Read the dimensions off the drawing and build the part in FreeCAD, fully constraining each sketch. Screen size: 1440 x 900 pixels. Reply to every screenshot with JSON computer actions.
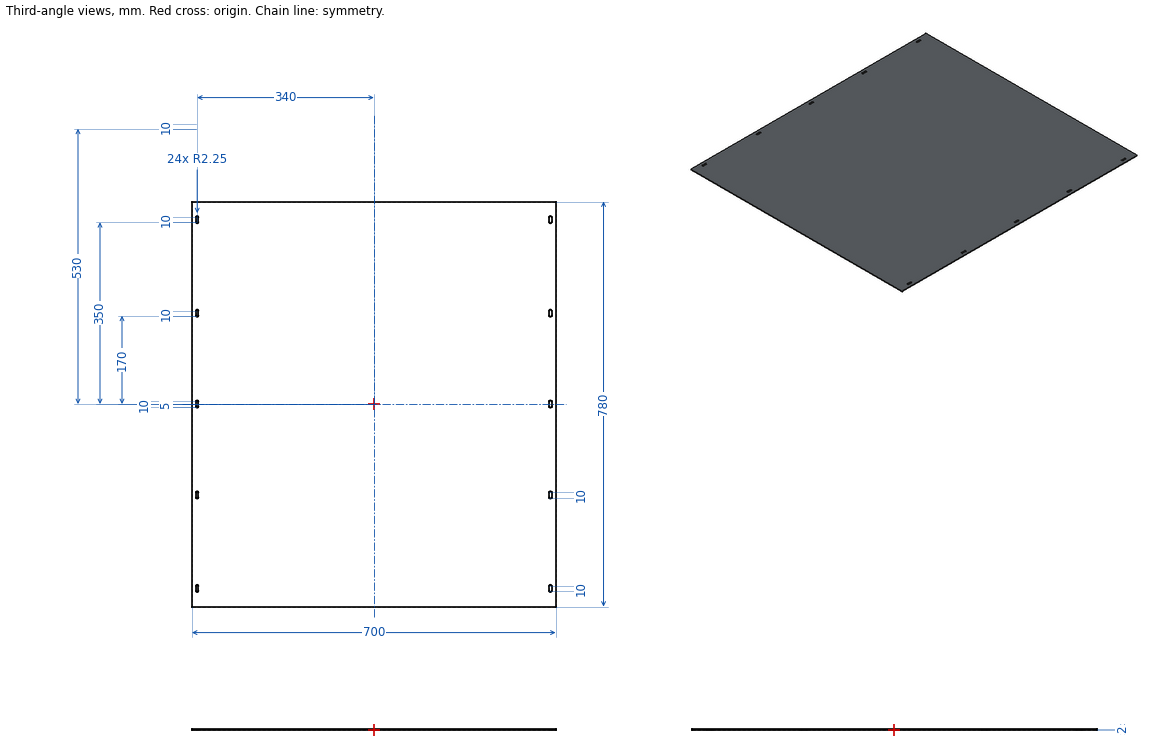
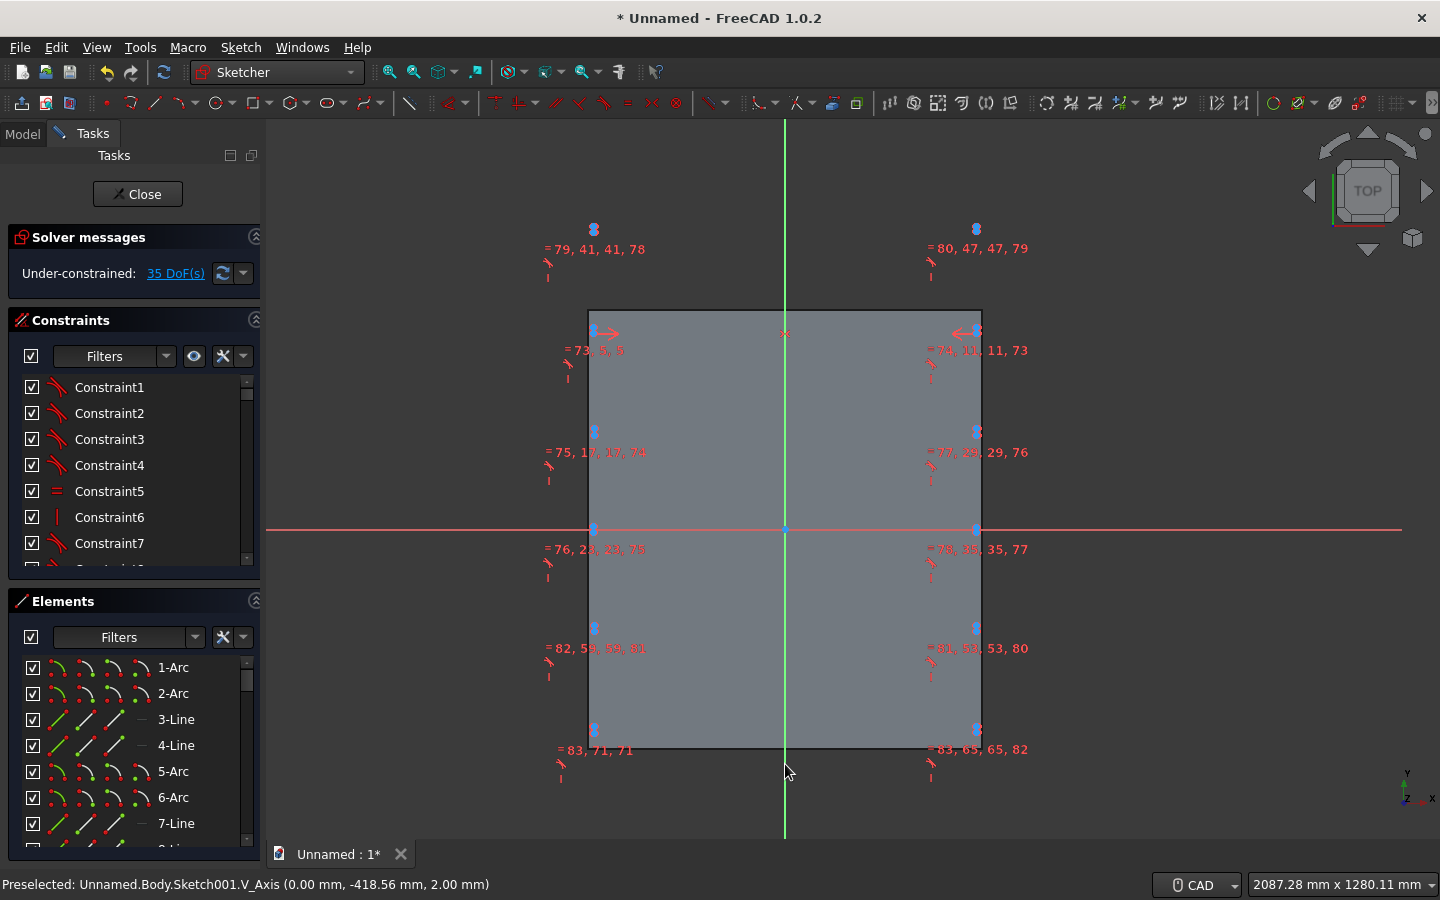
{"action": "scroll", "coordinate": [594, 435], "scroll_direction": "up", "scroll_amount": 12}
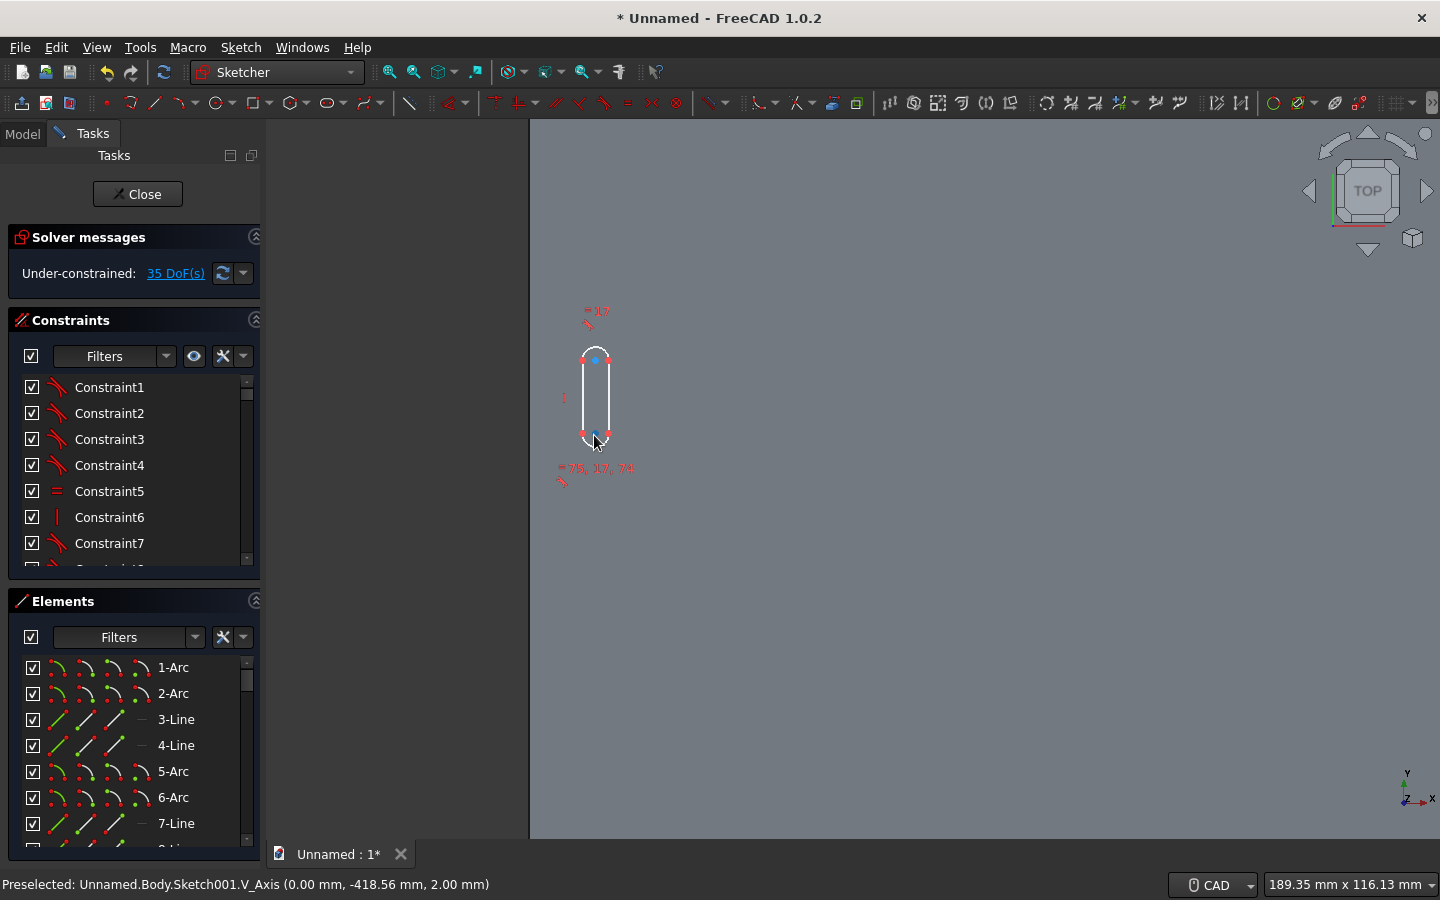
{"action": "left_click", "coordinate": [596, 434]}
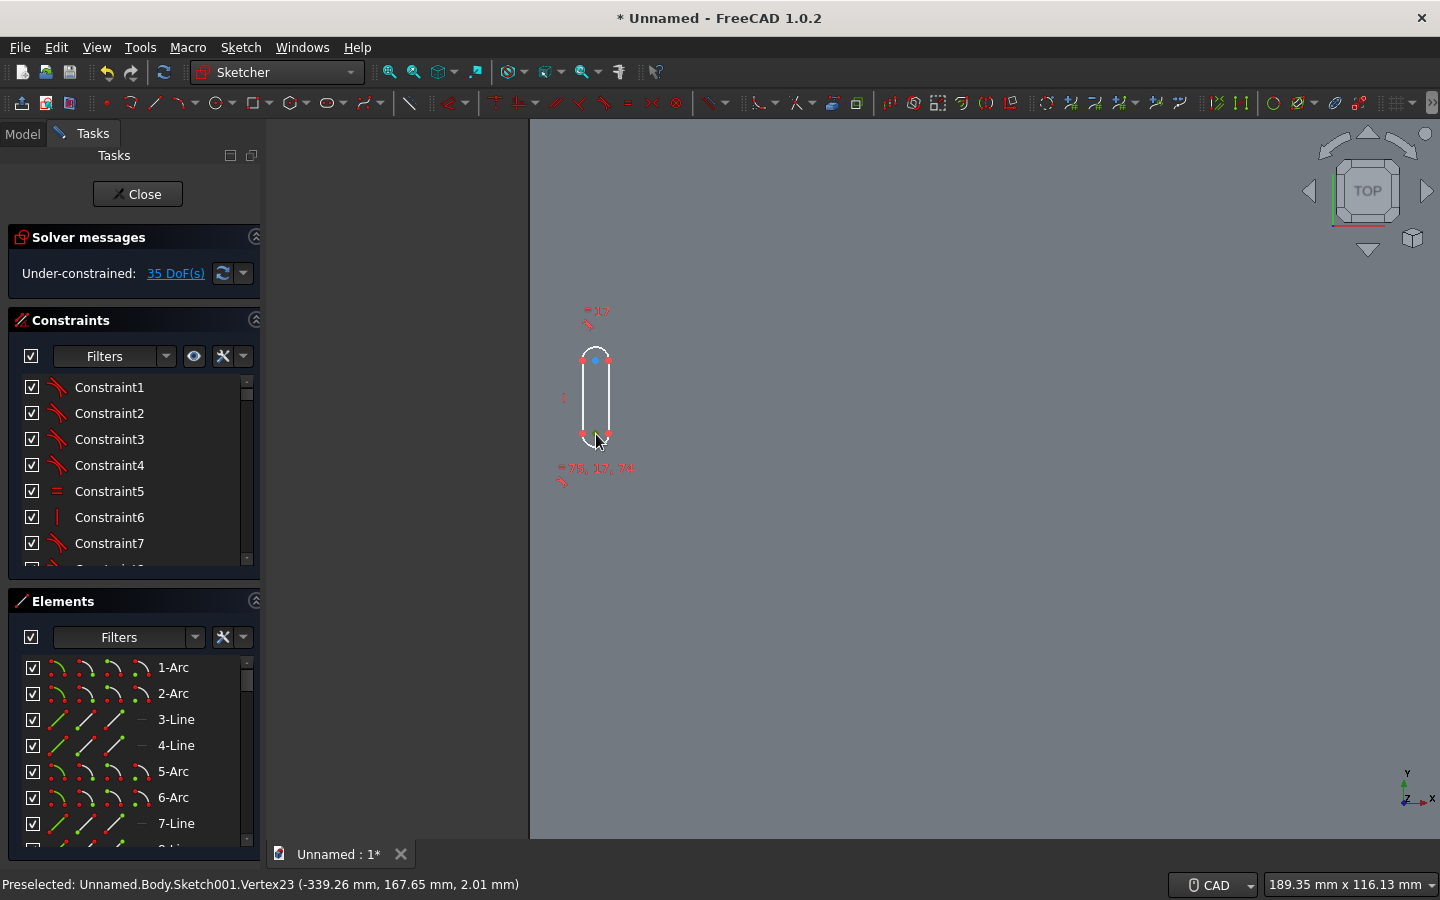
{"action": "scroll", "coordinate": [593, 435], "scroll_direction": "down", "scroll_amount": 12}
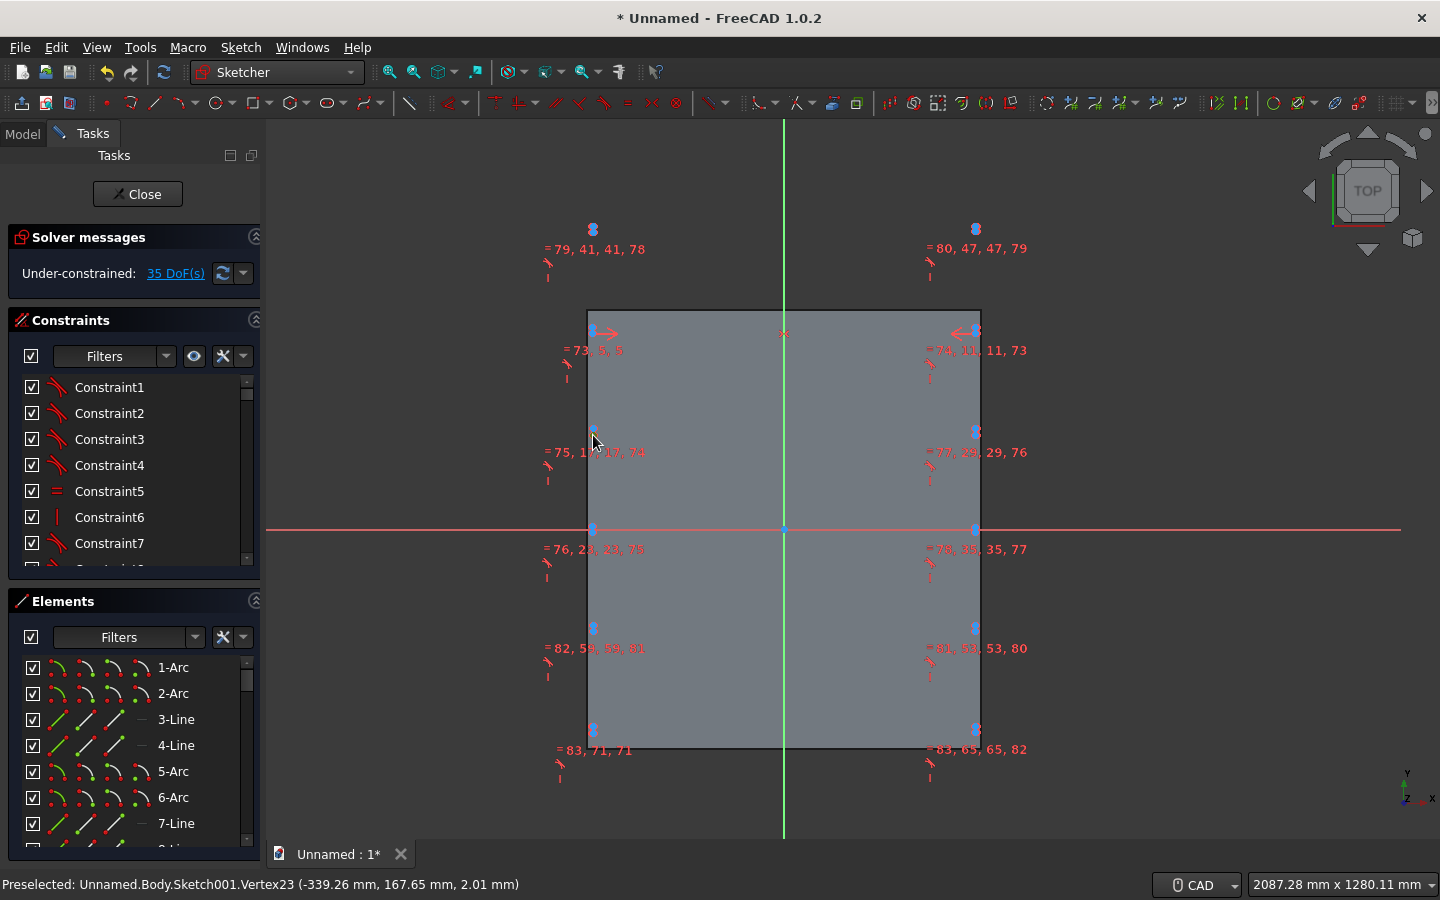
{"action": "scroll", "coordinate": [976, 435], "scroll_direction": "up", "scroll_amount": 12}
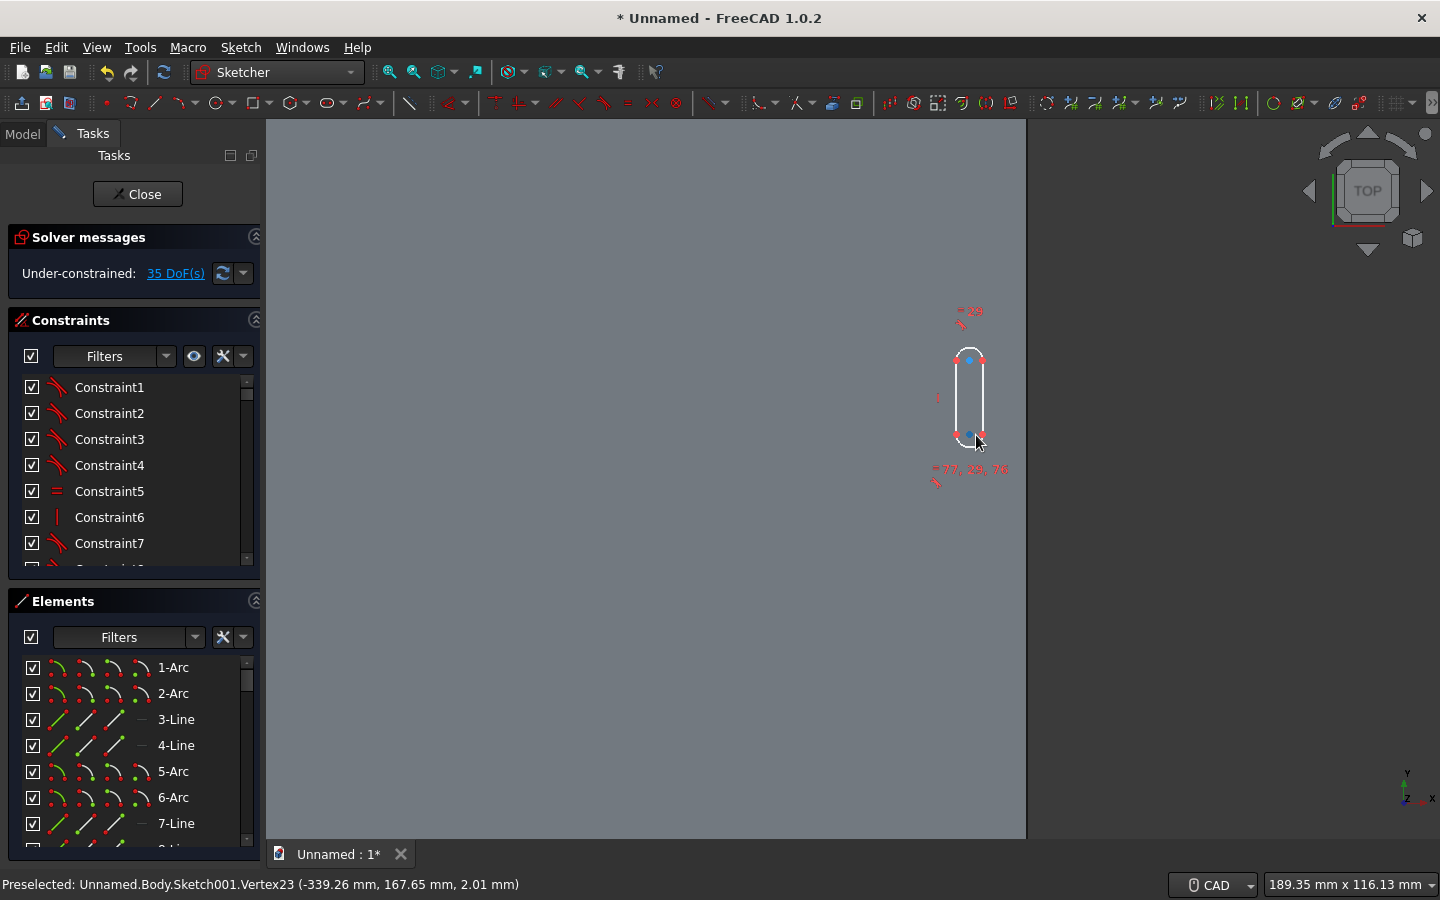
{"action": "left_click", "coordinate": [970, 434]}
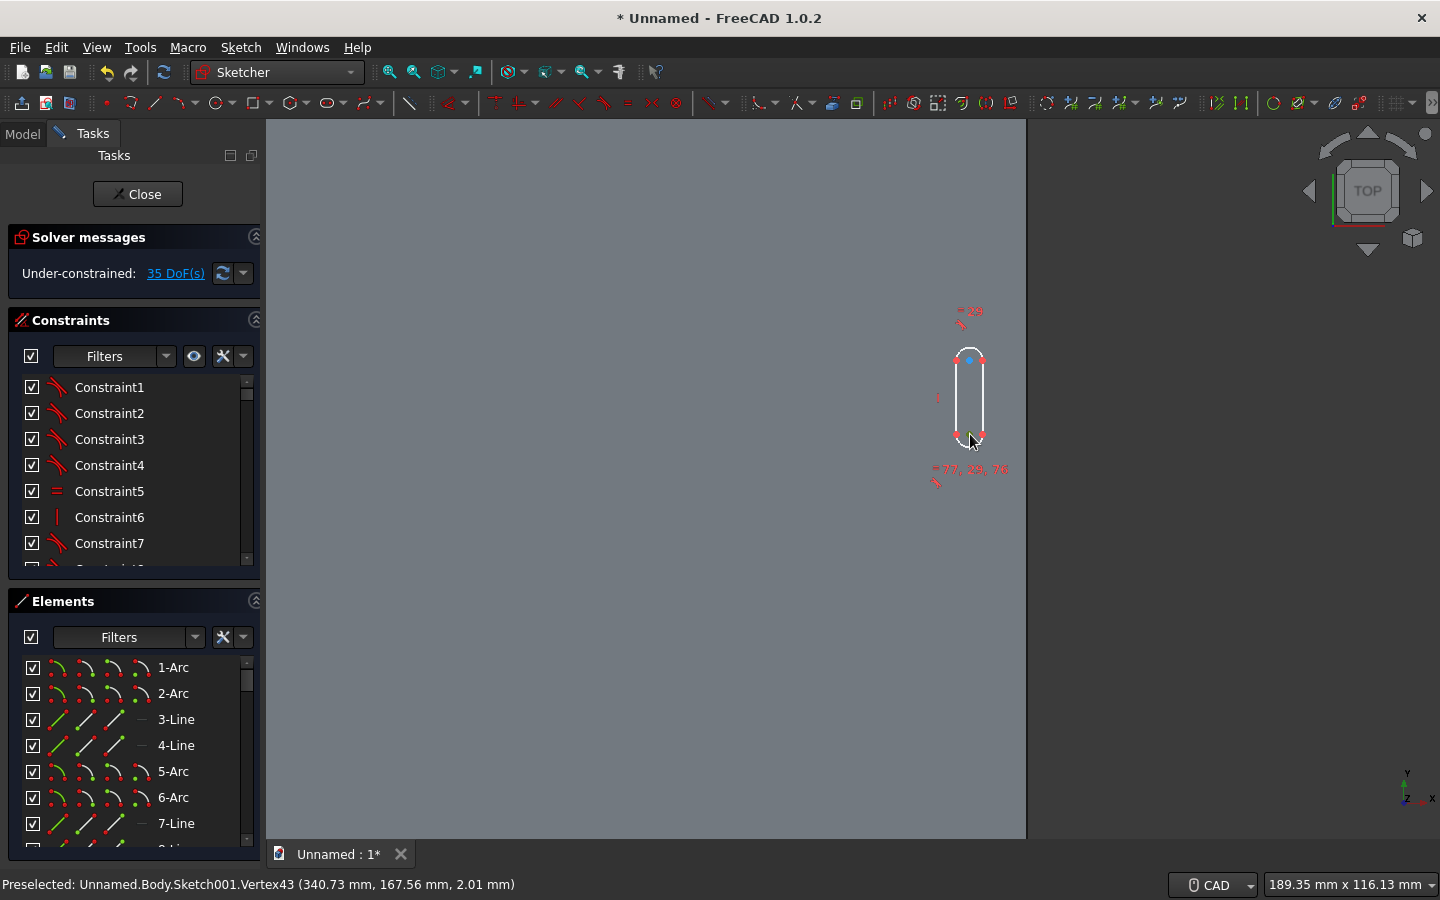
{"action": "scroll", "coordinate": [977, 435], "scroll_direction": "down", "scroll_amount": 12}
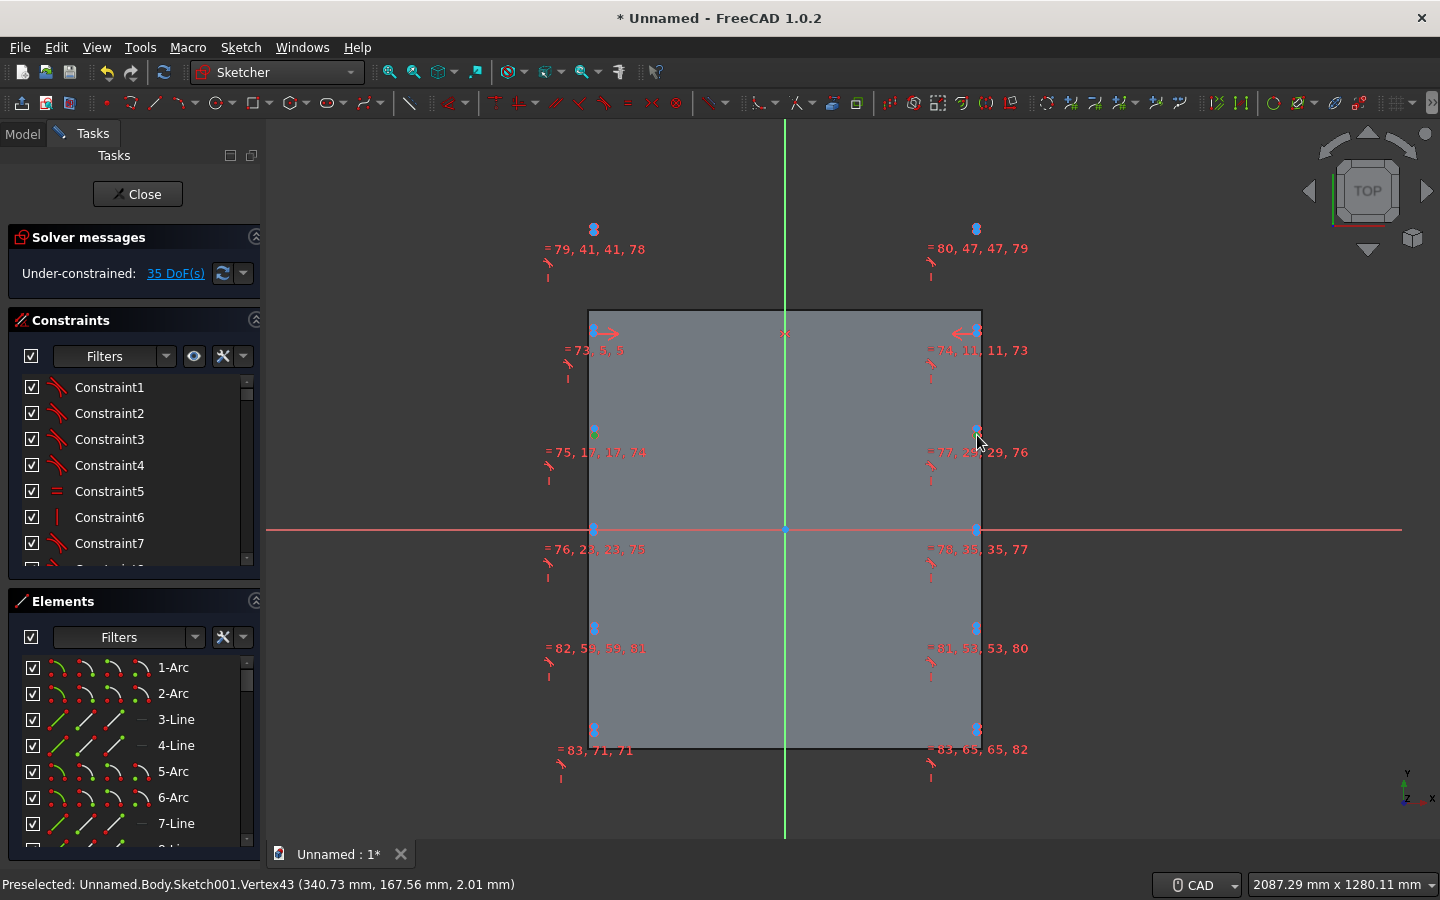
{"action": "left_click", "coordinate": [785, 764]}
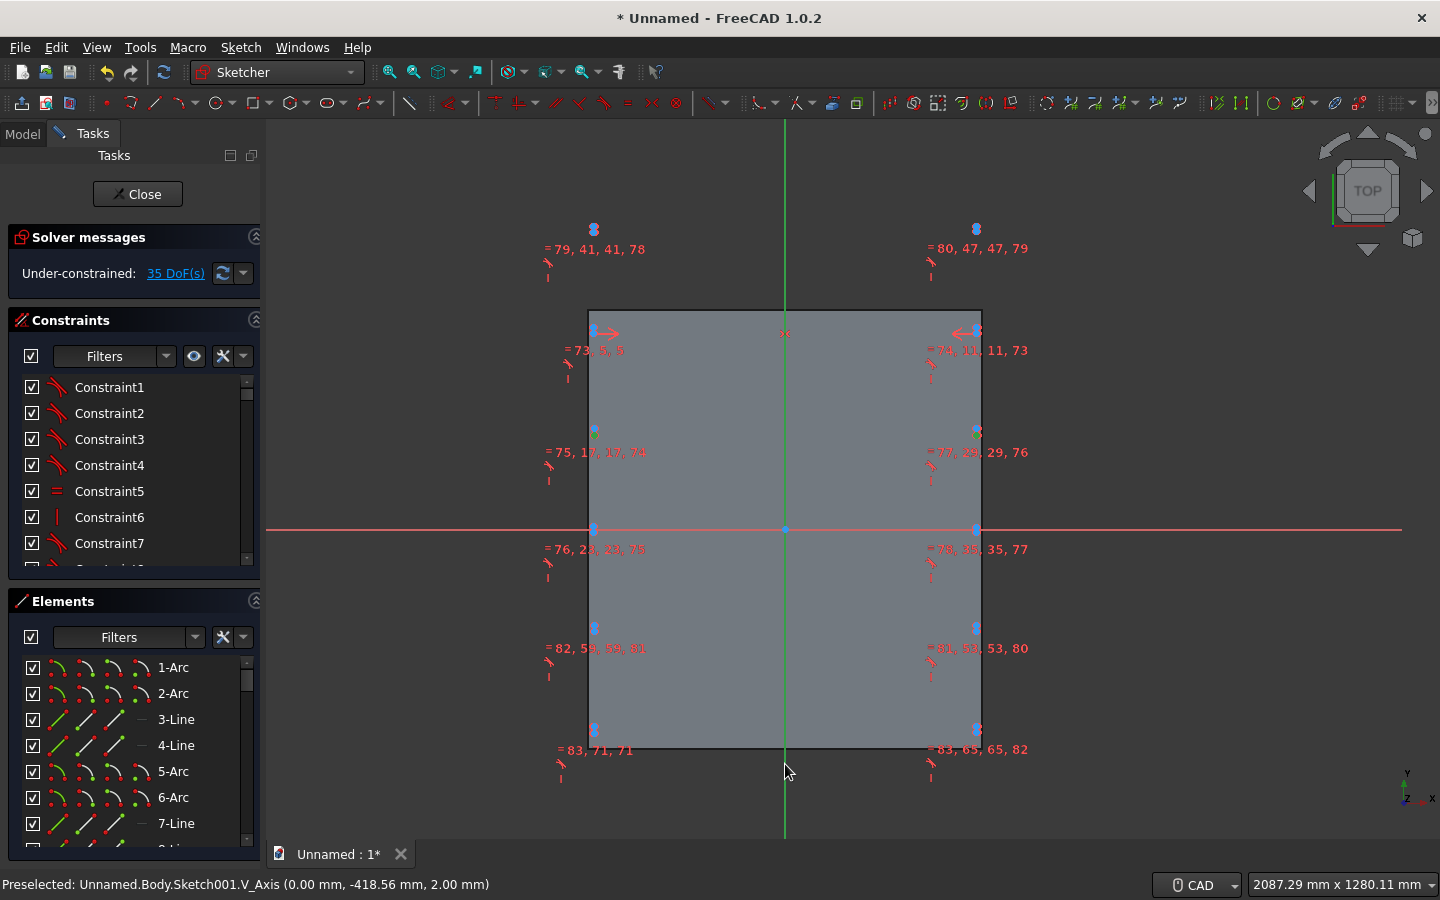
{"action": "key", "text": "s"}